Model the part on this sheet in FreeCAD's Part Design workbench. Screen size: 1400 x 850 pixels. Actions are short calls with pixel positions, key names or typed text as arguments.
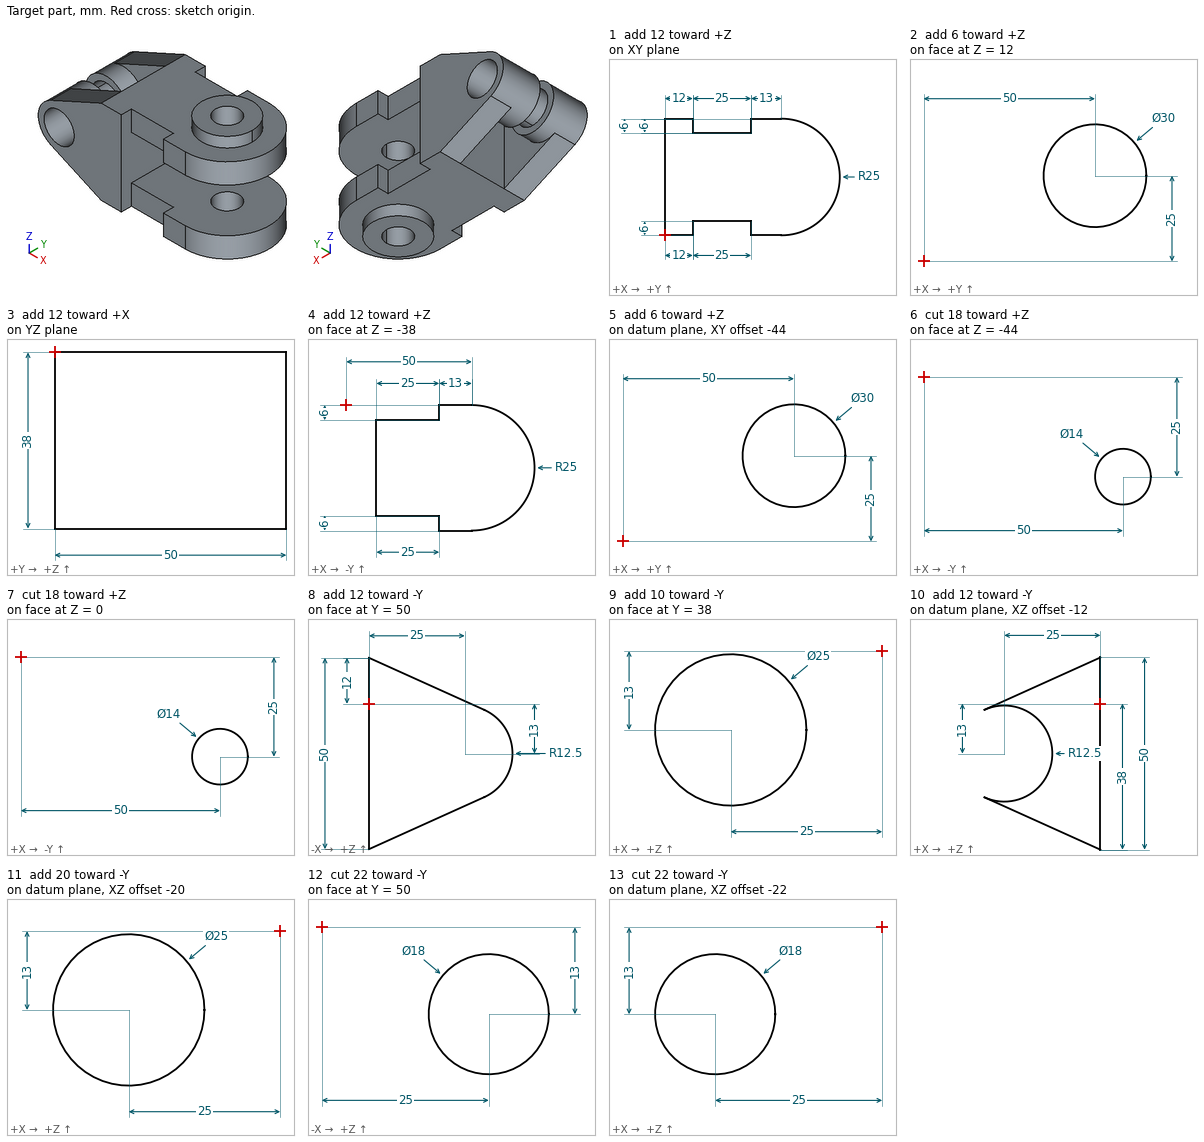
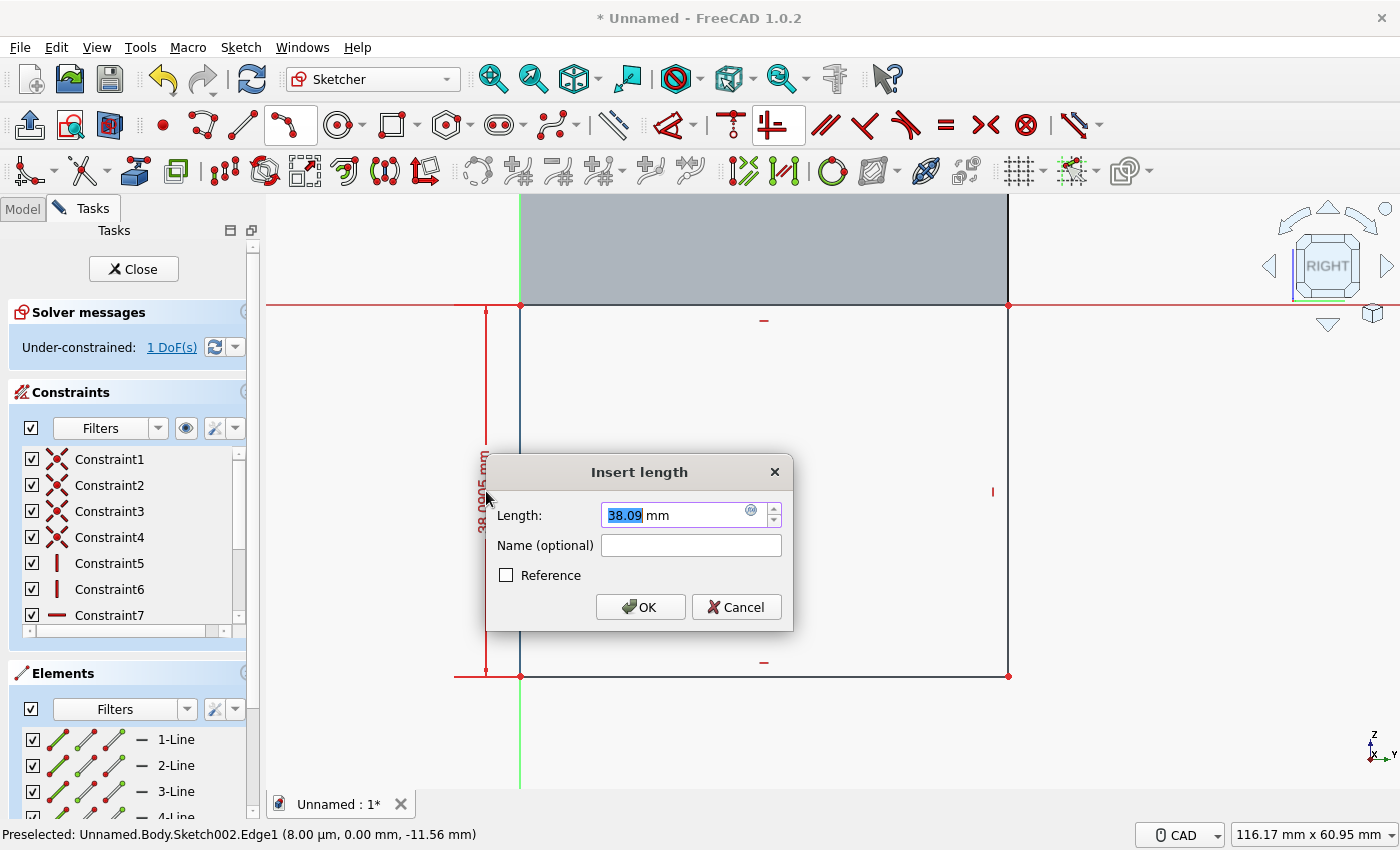
text(38)
key(Return)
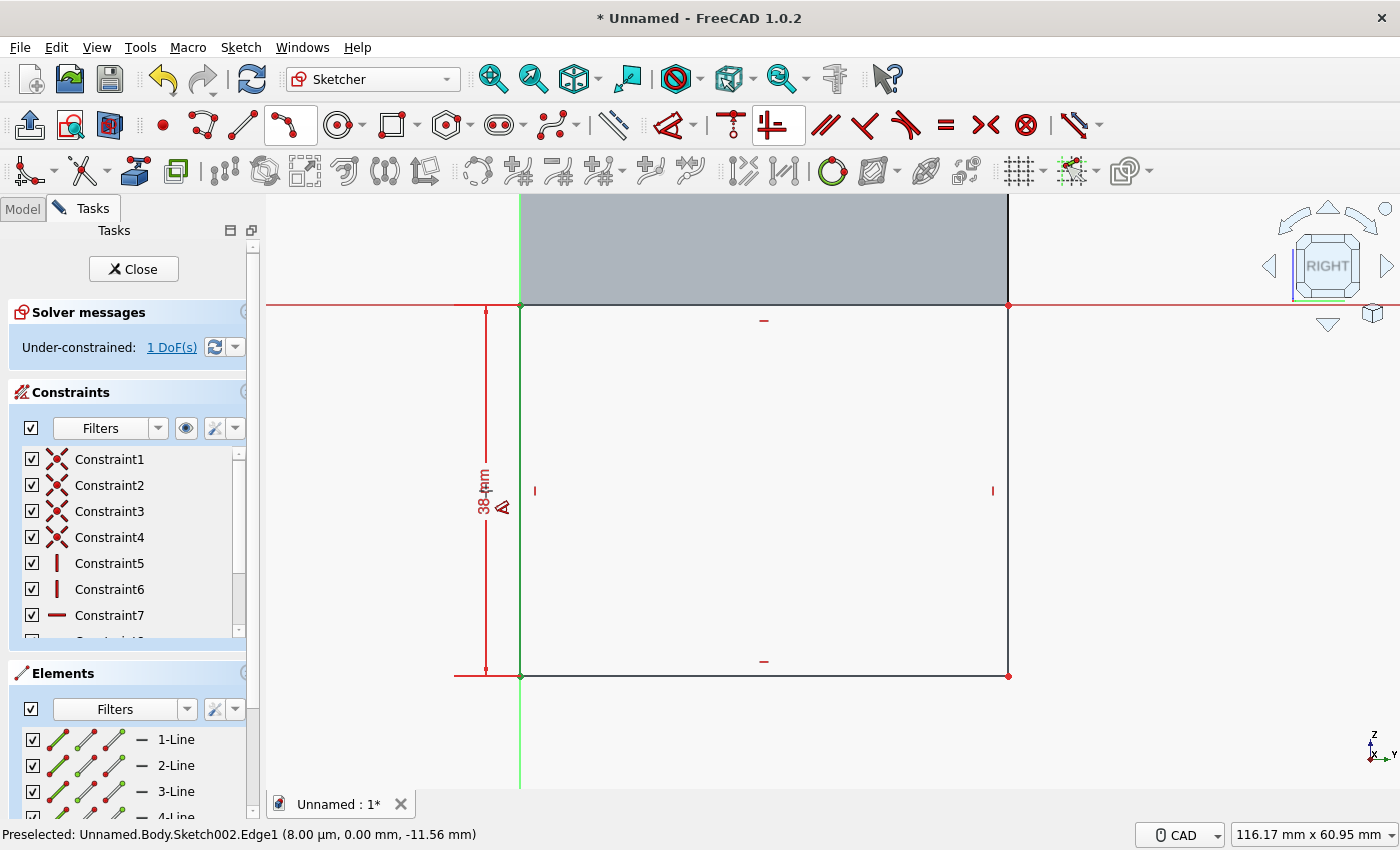
click(667, 676)
click(764, 710)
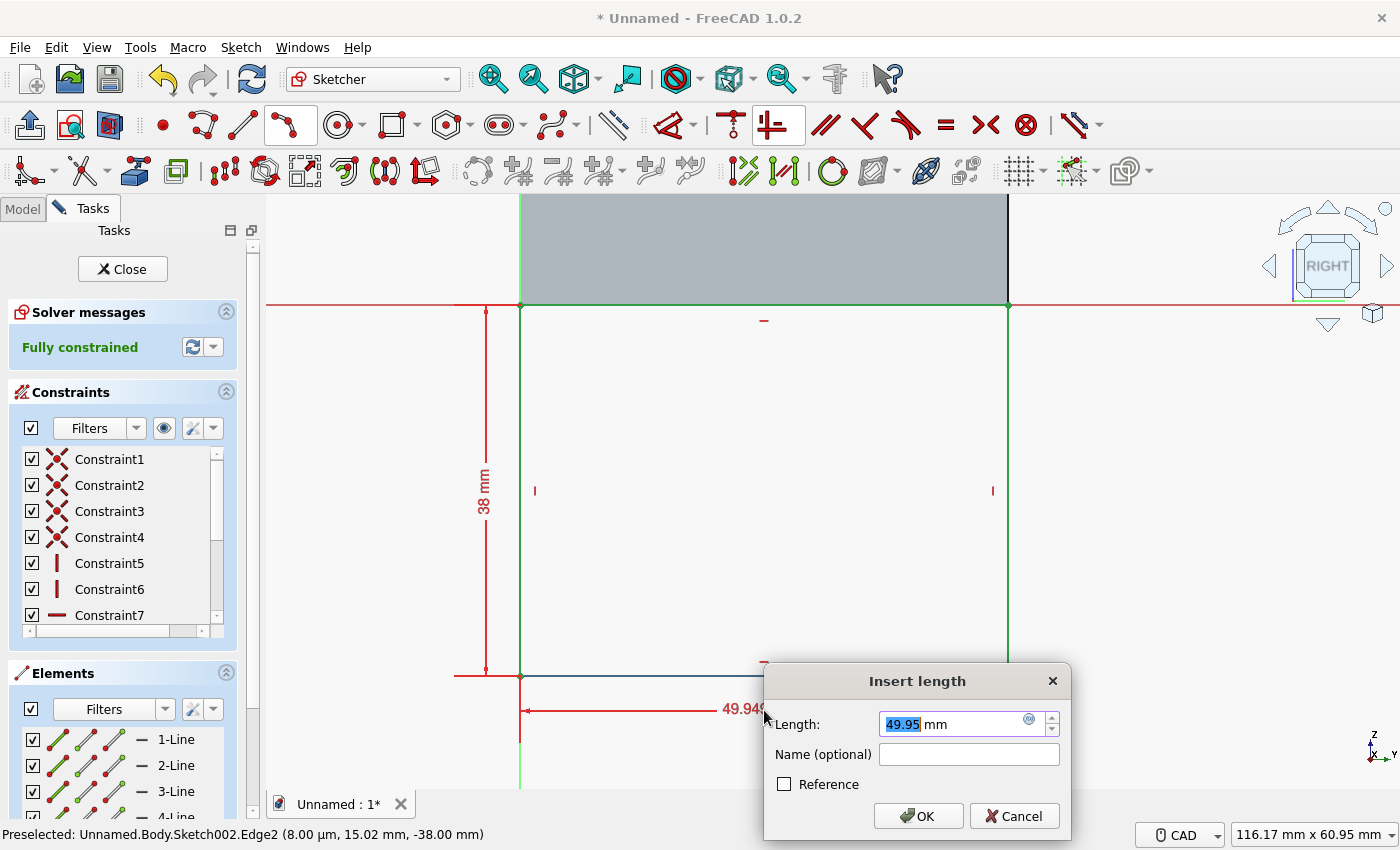
text(50)
key(Return)
key(Escape)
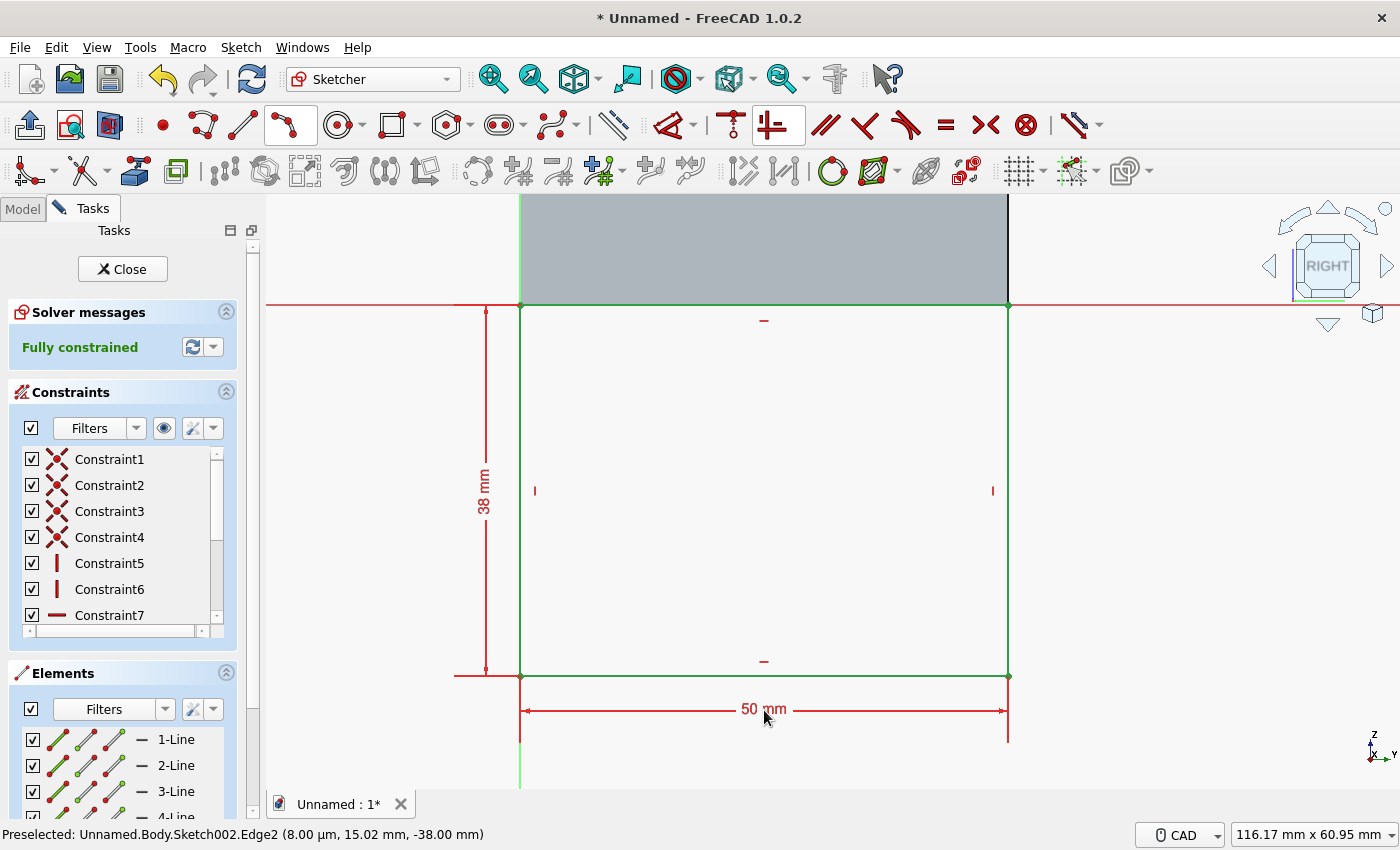
click(123, 269)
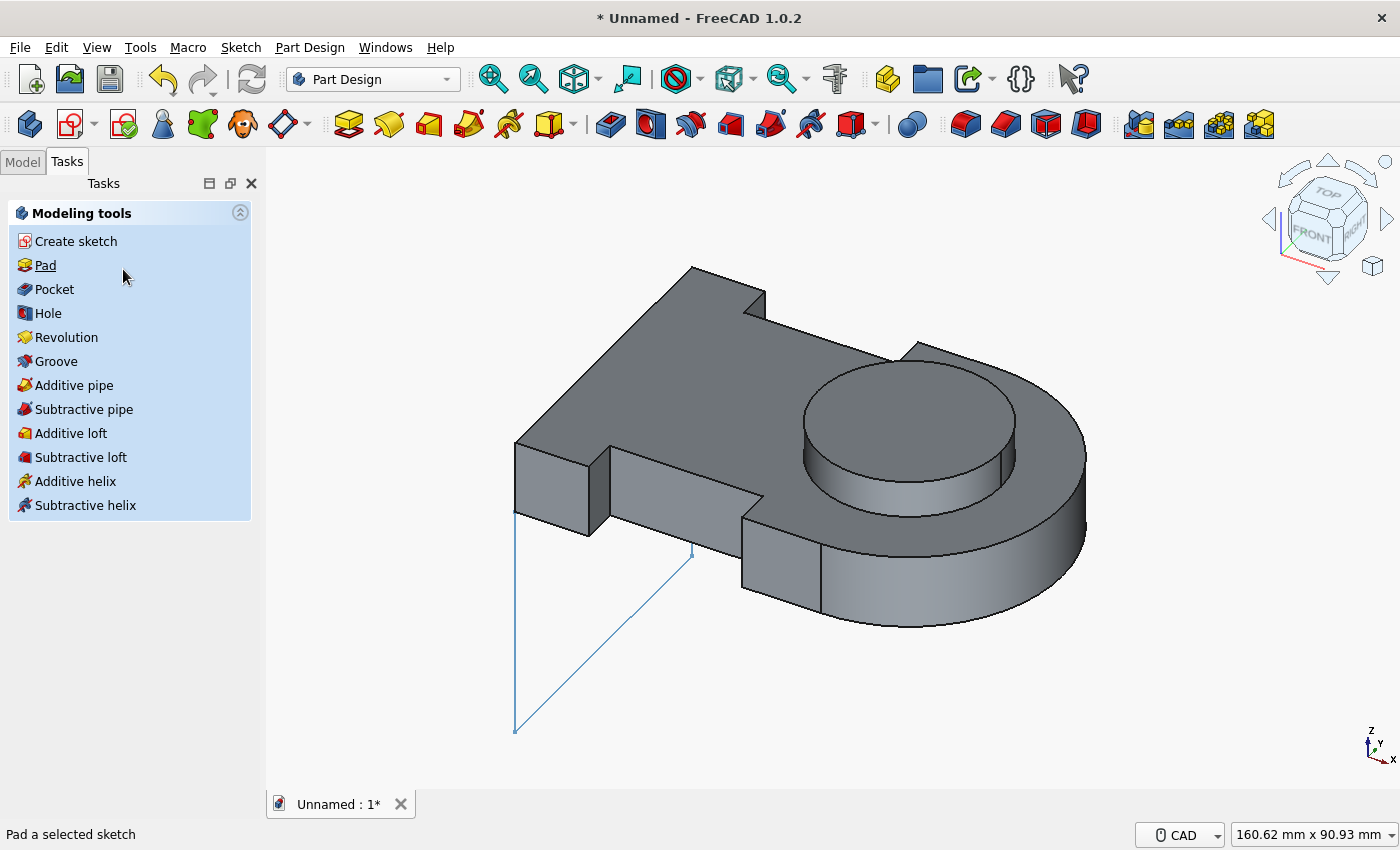
click(350, 124)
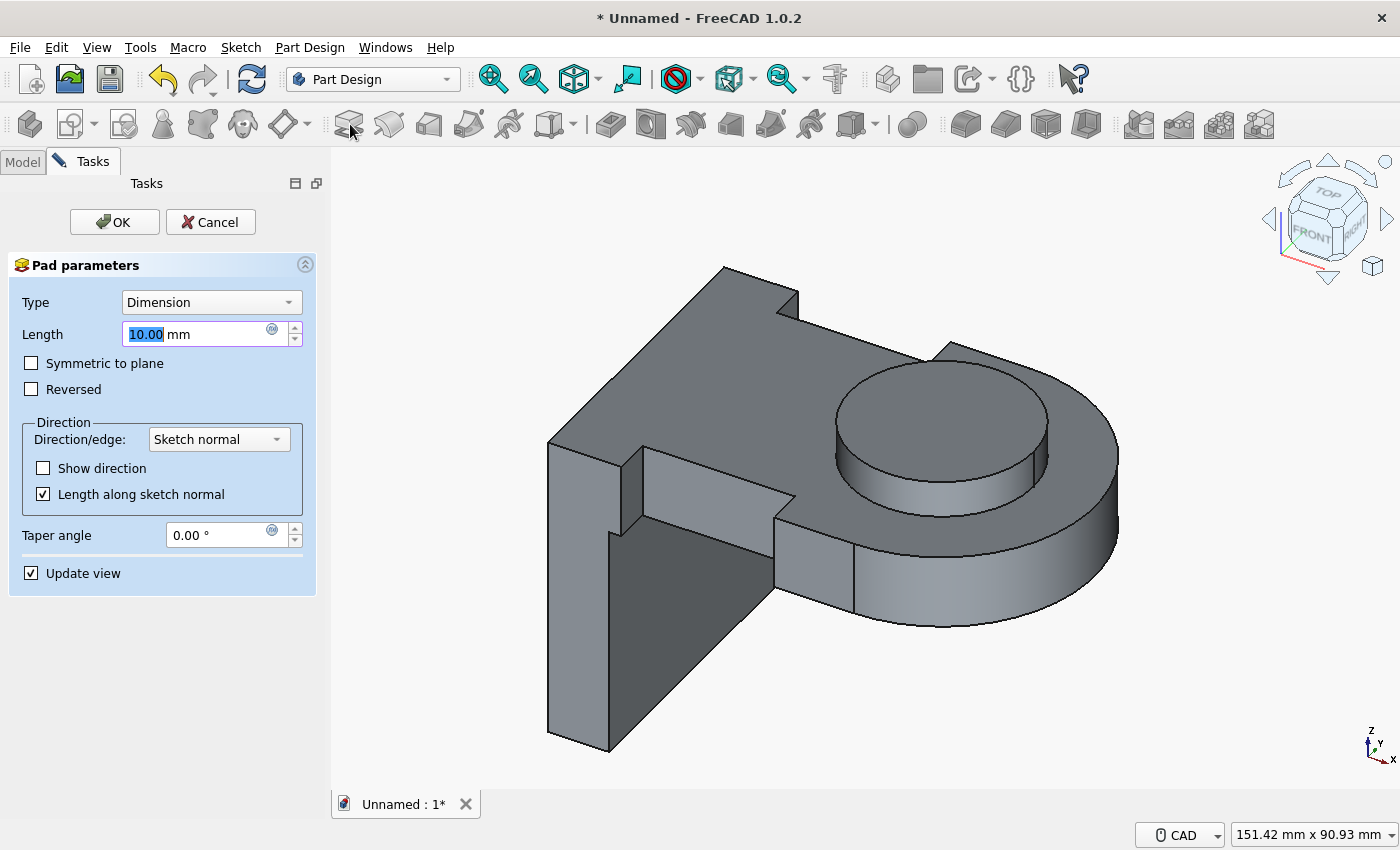
text(12)
key(Tab)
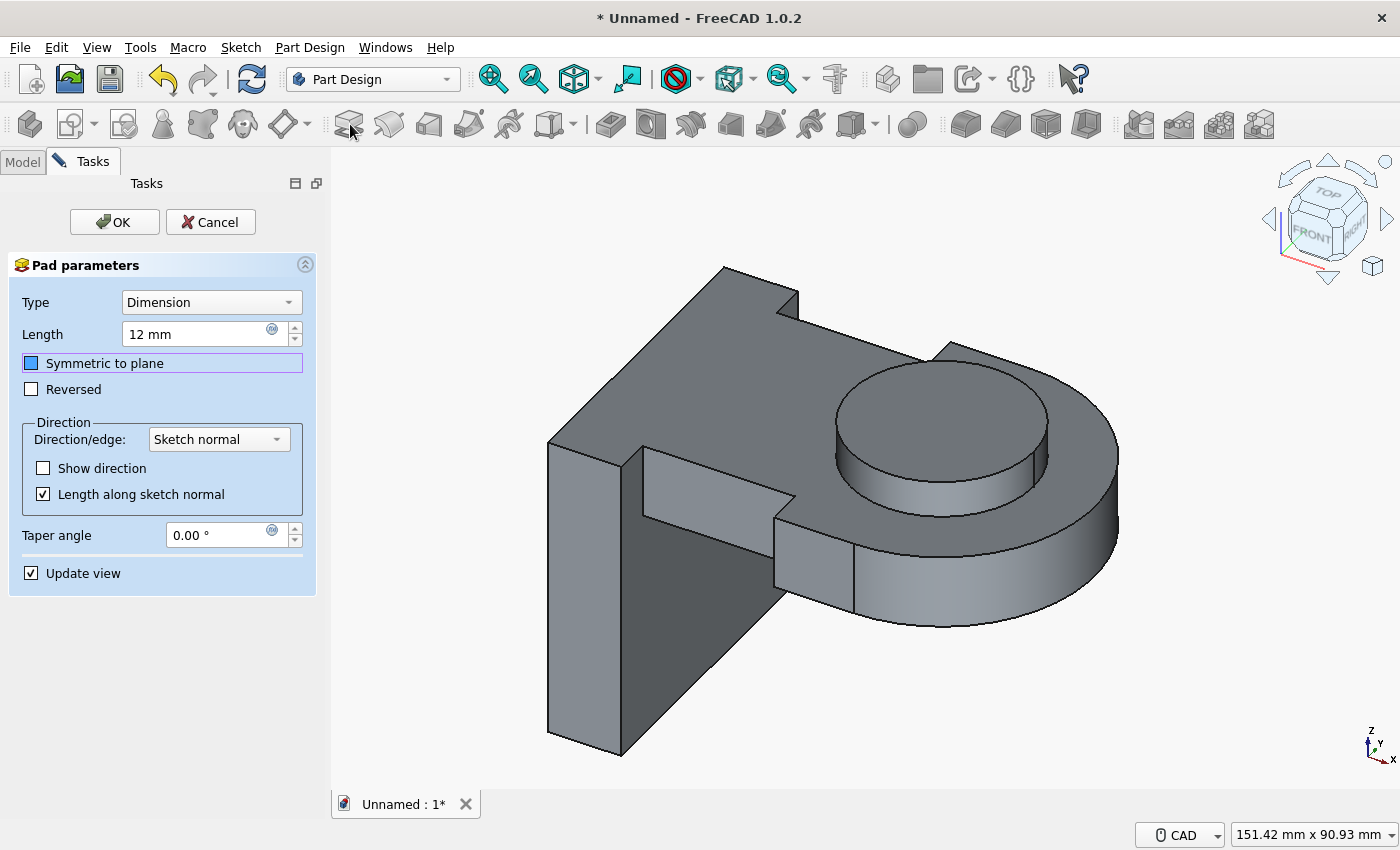
click(115, 222)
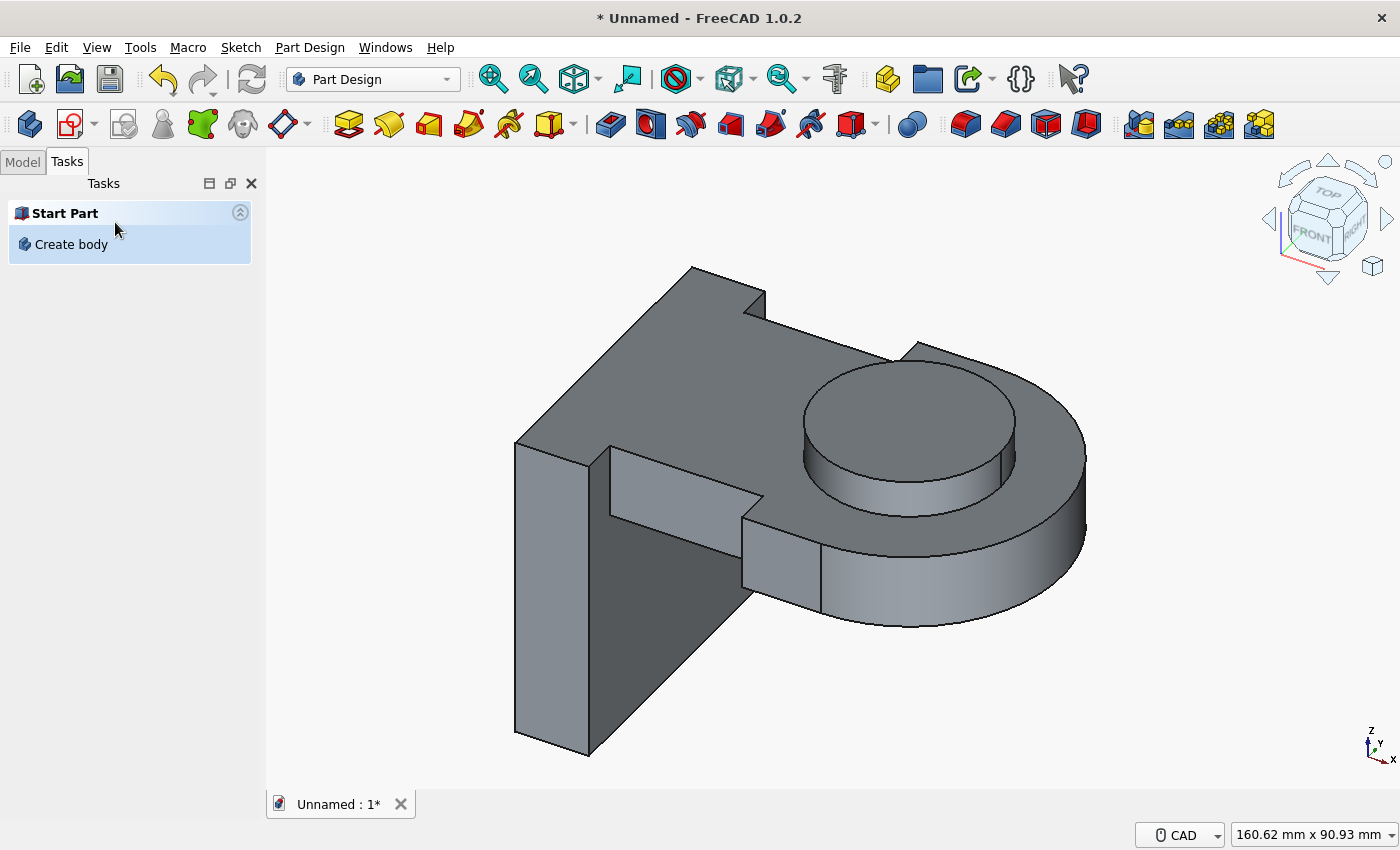
click(494, 80)